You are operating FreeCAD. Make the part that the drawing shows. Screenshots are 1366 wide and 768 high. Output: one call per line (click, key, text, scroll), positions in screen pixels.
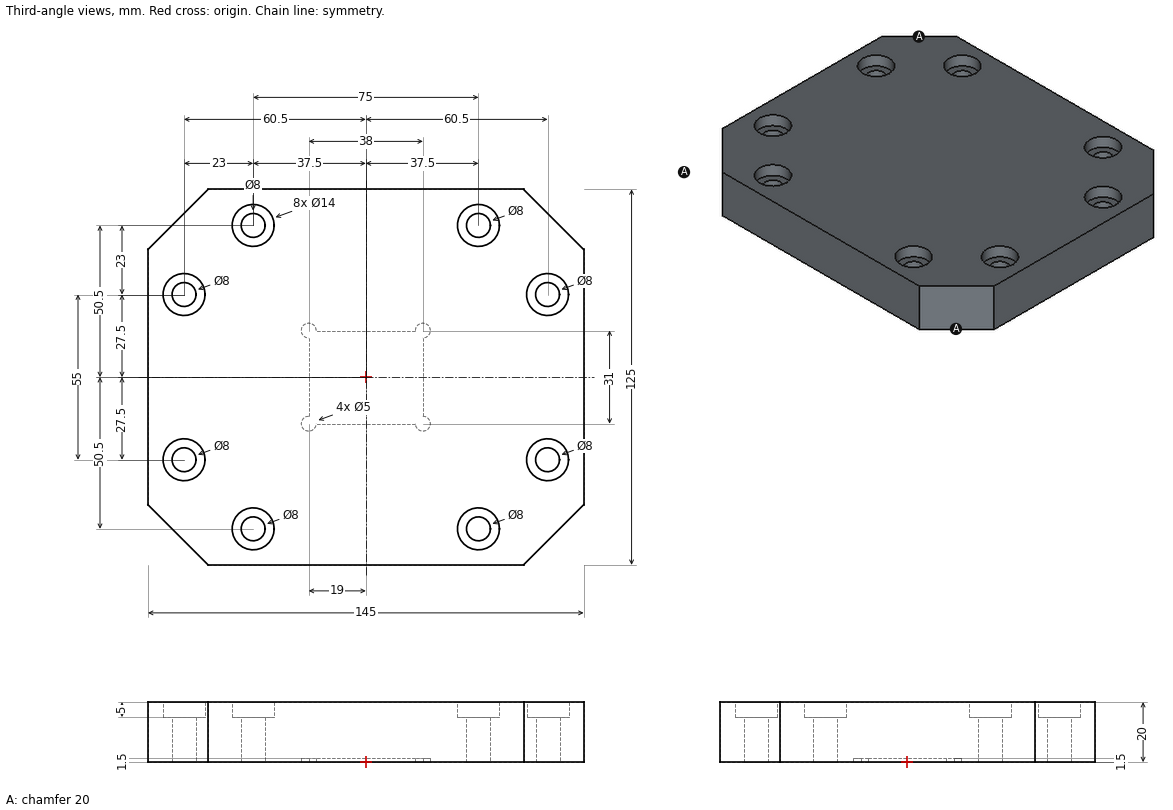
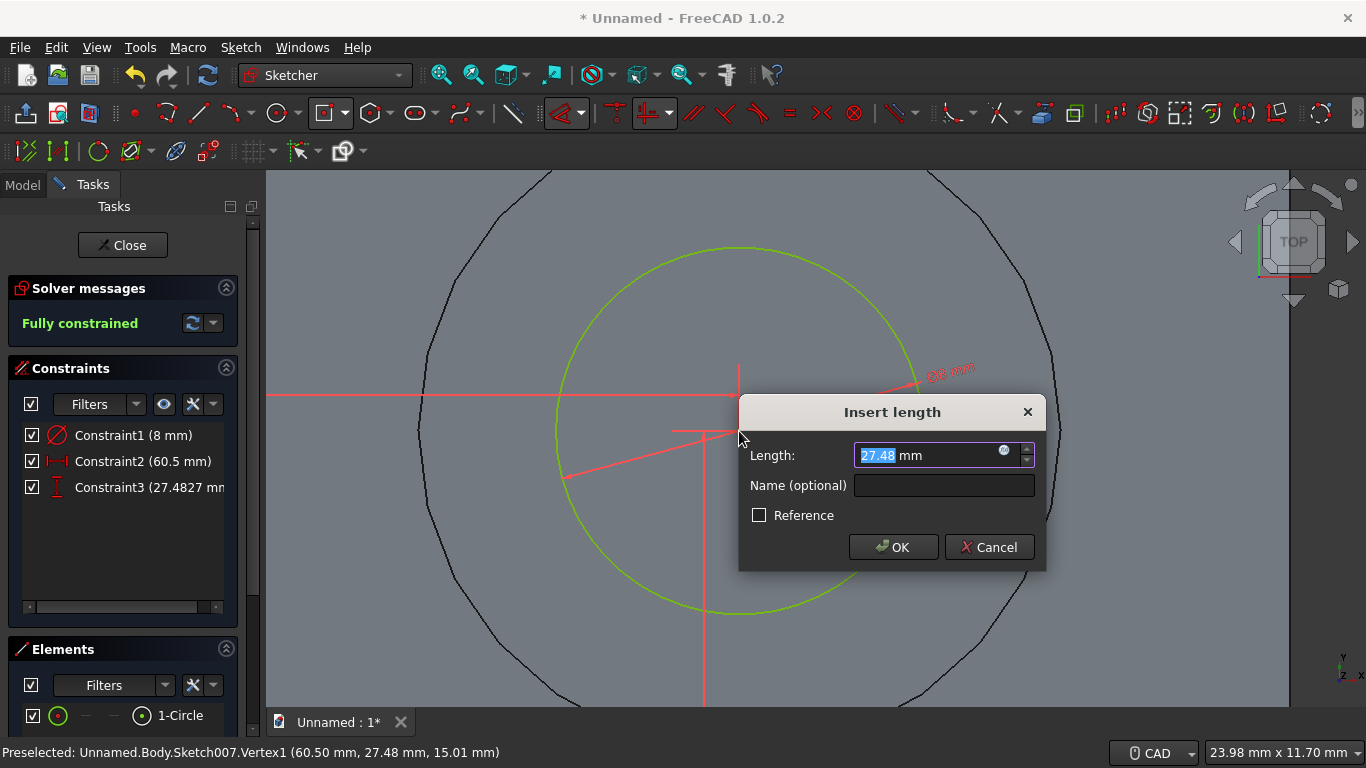
text(27.5)
key(Return)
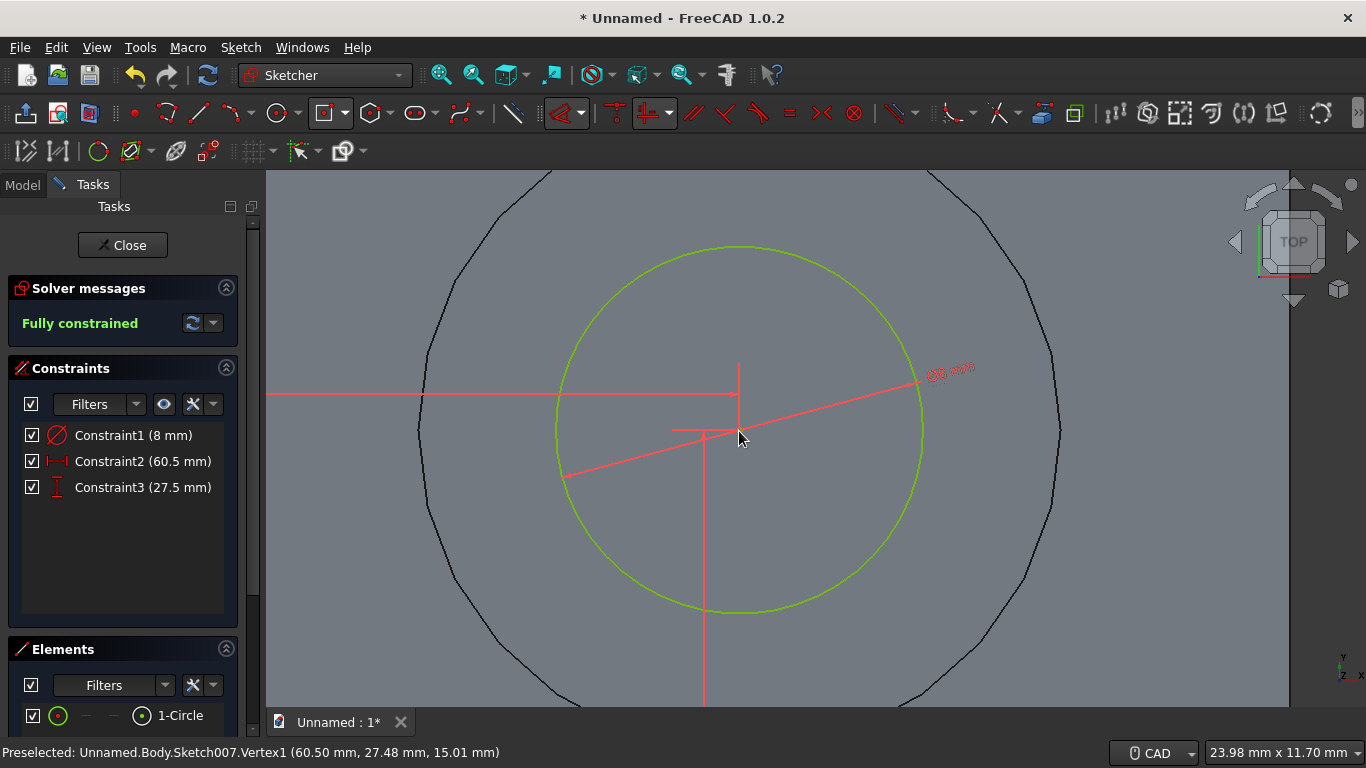
click(123, 245)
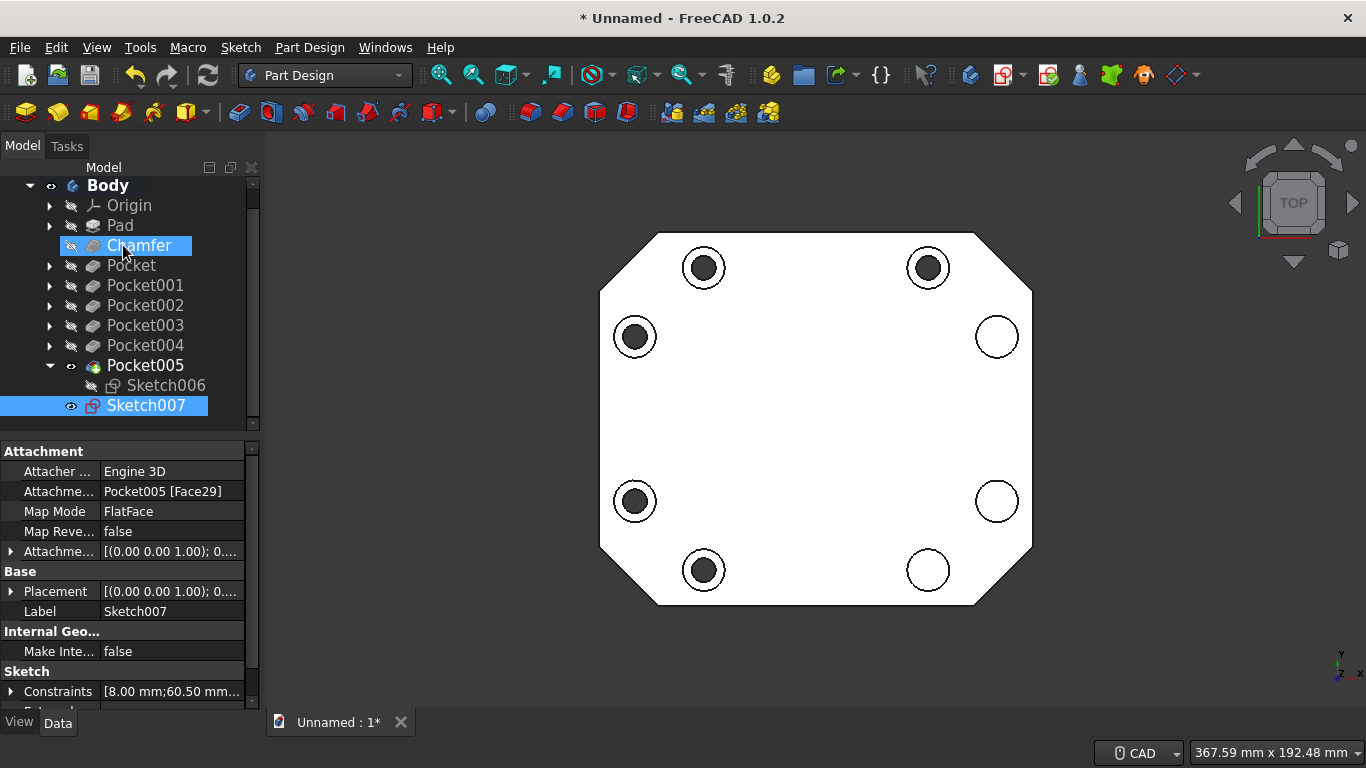
click(240, 112)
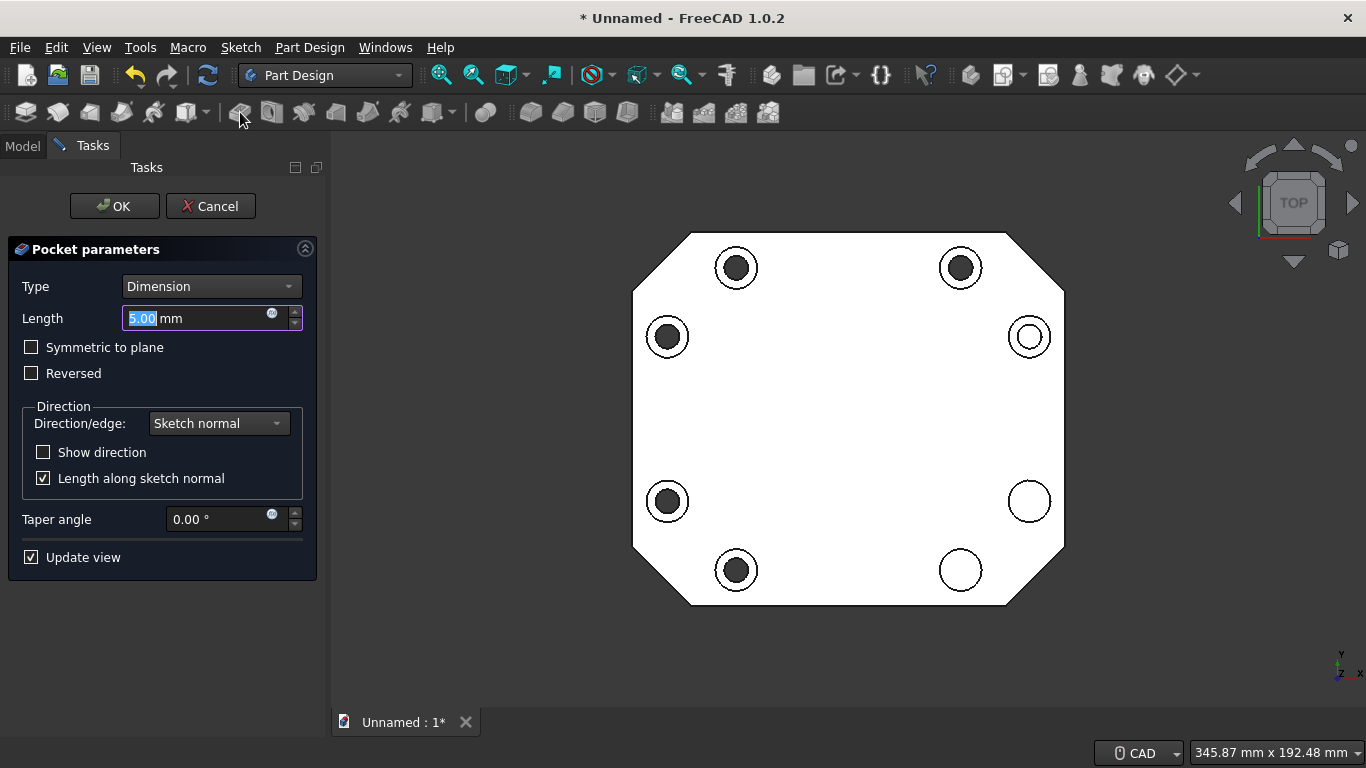
click(212, 286)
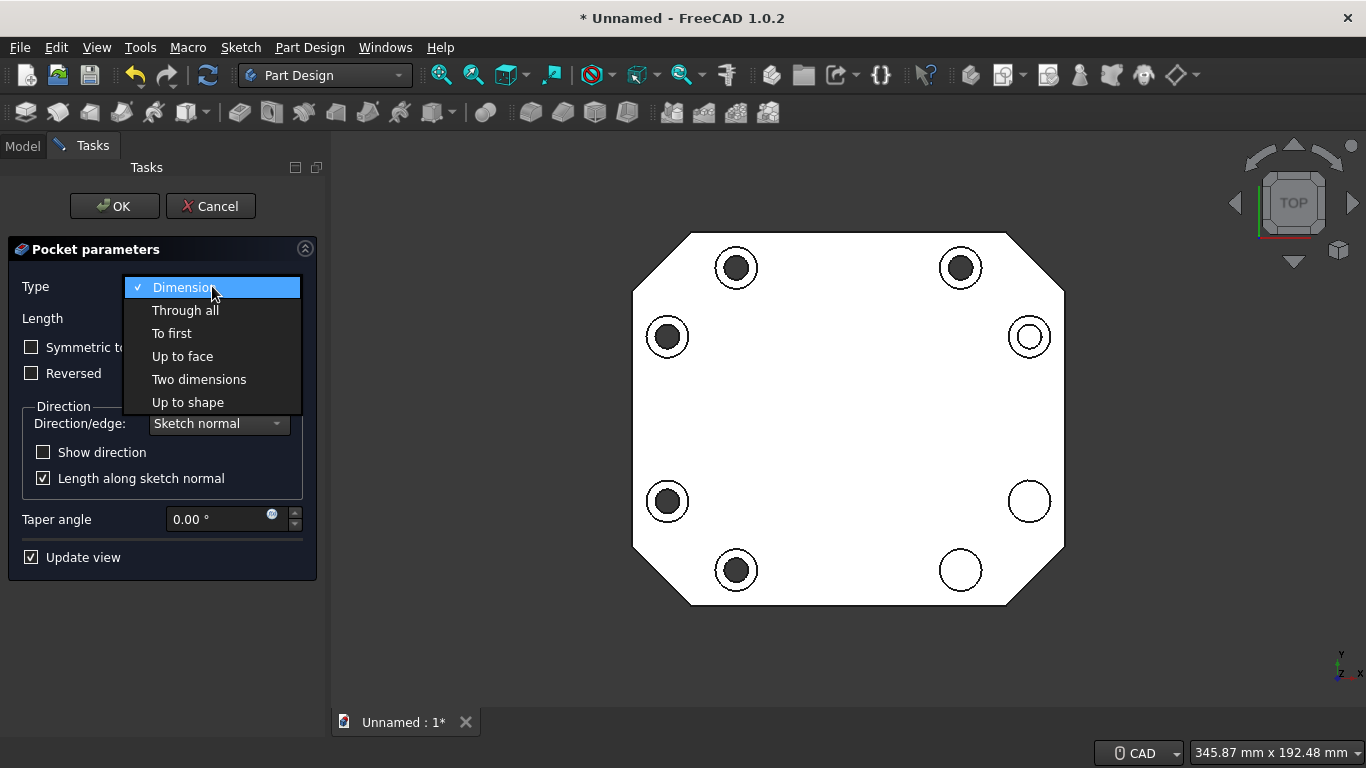
click(212, 334)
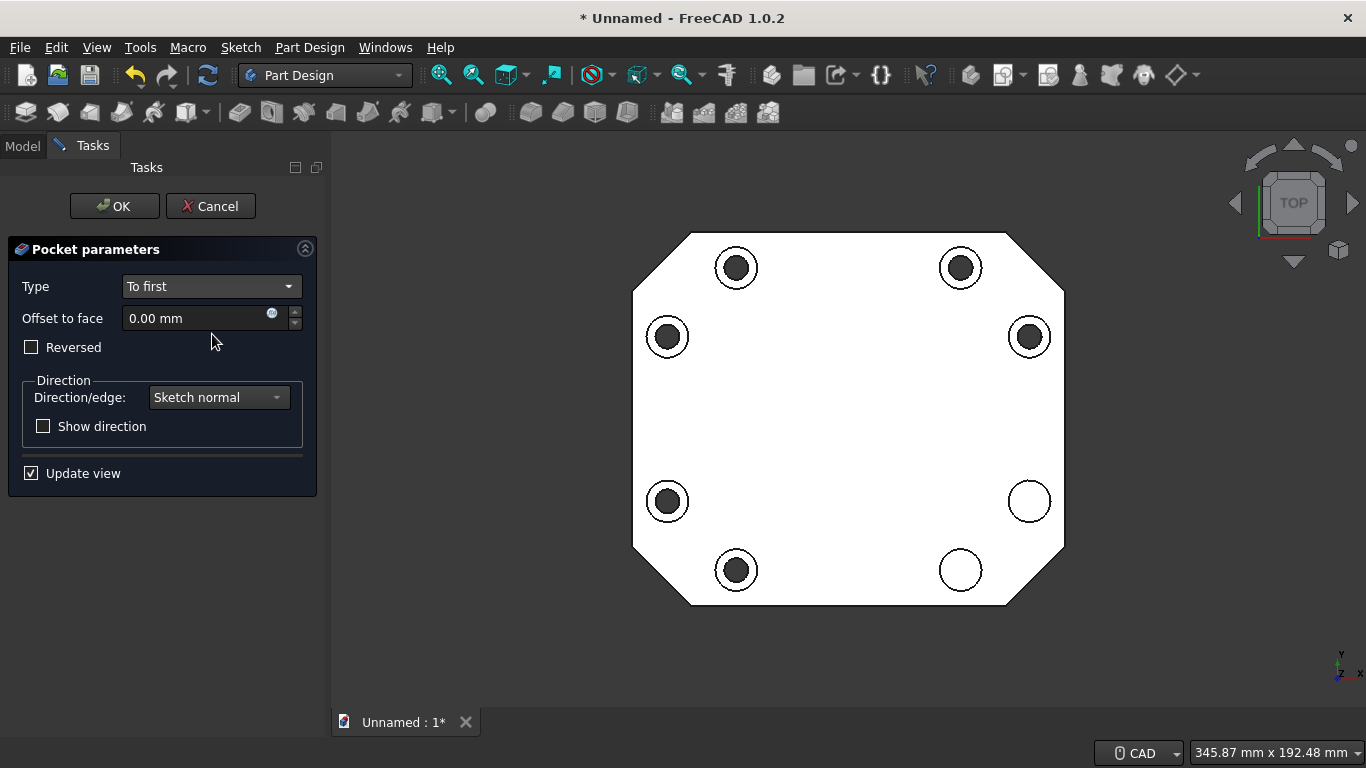
click(115, 206)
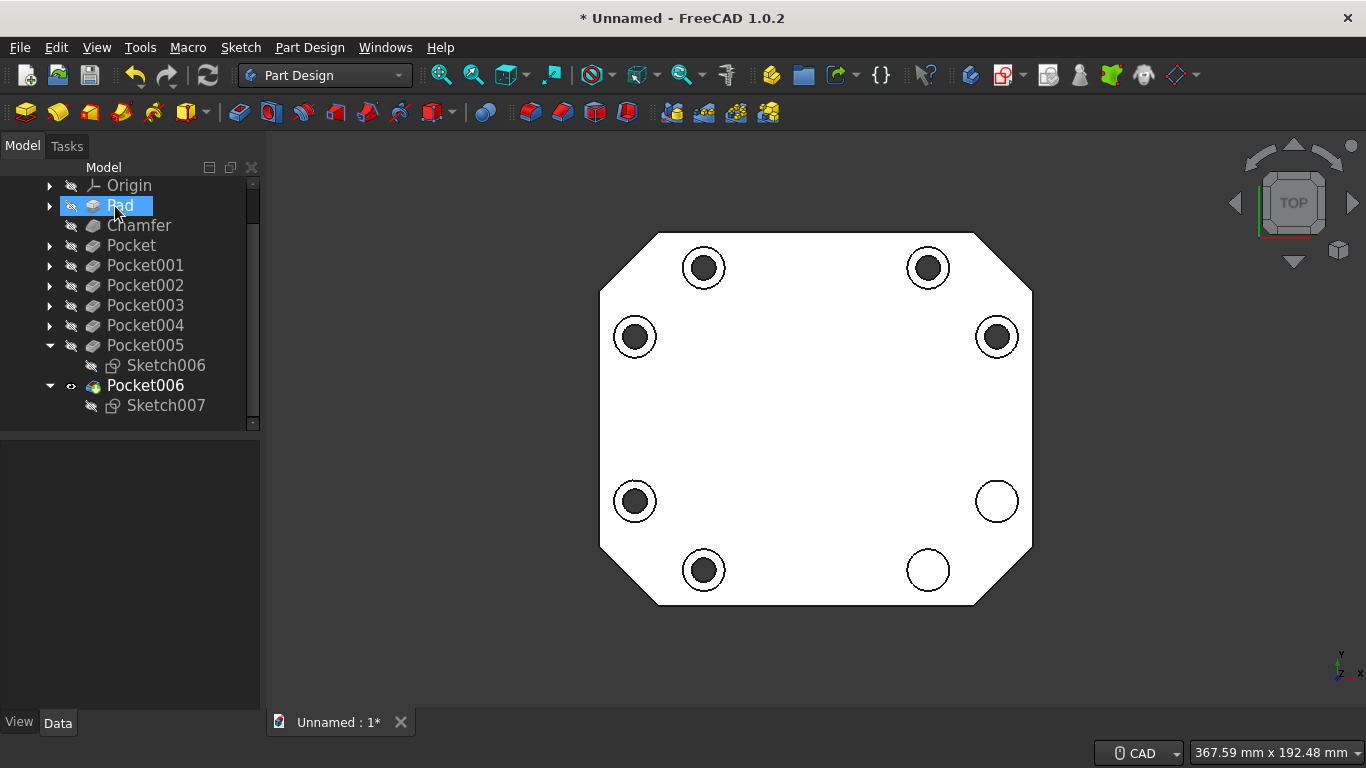
click(928, 569)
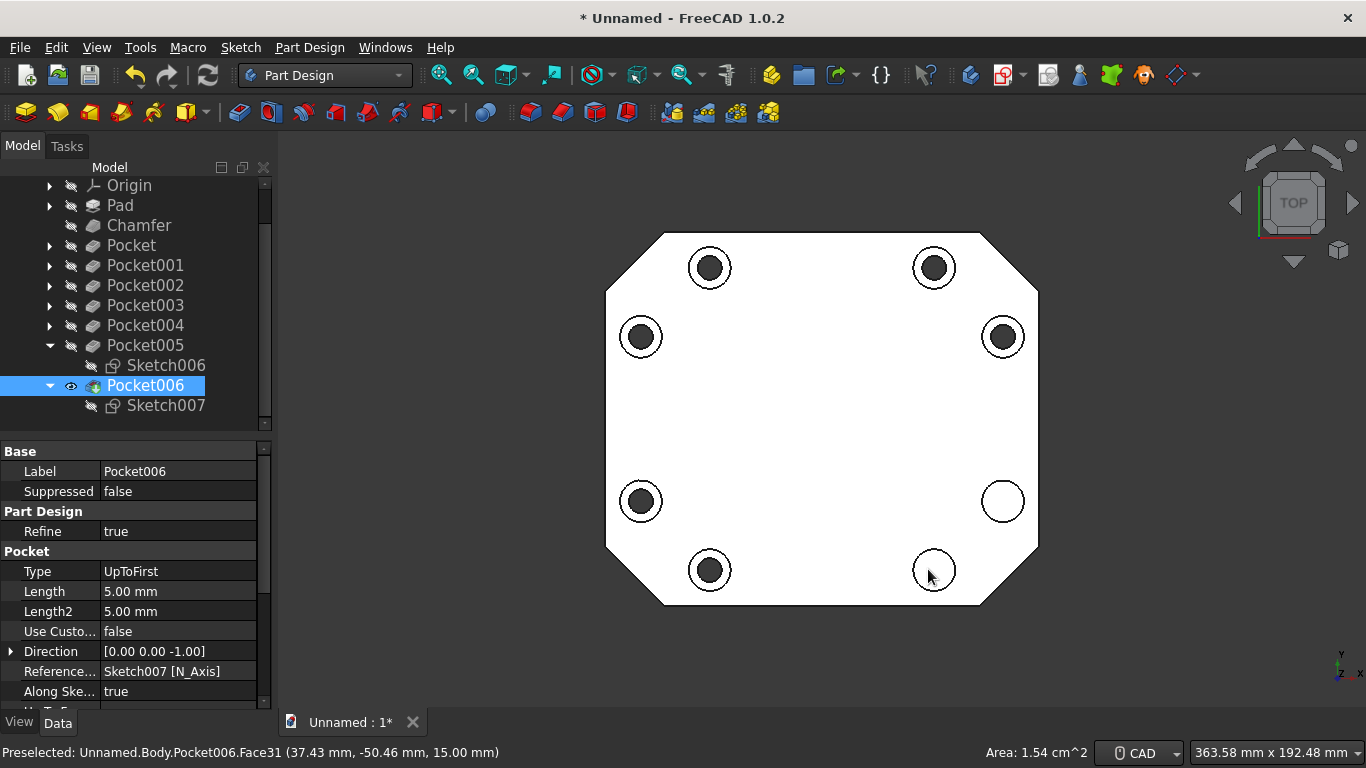
click(1004, 76)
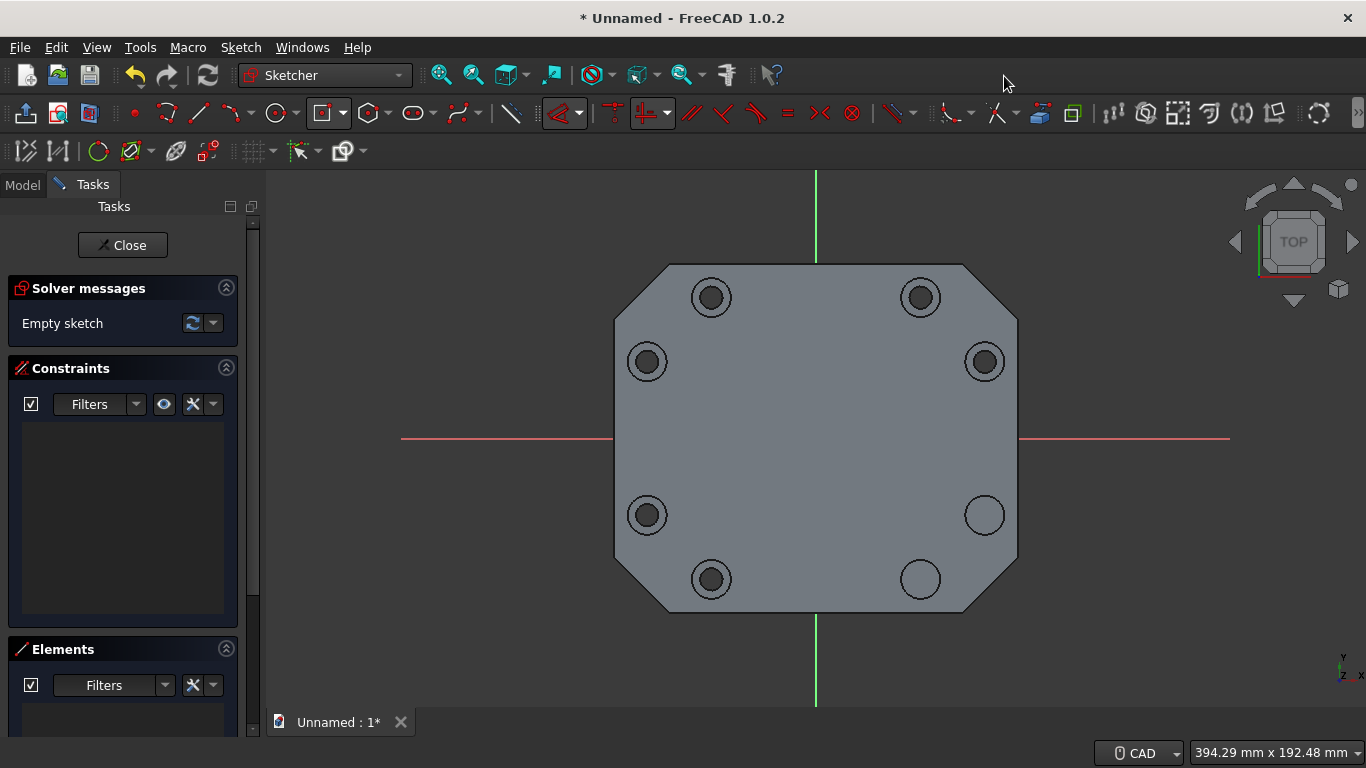
click(90, 114)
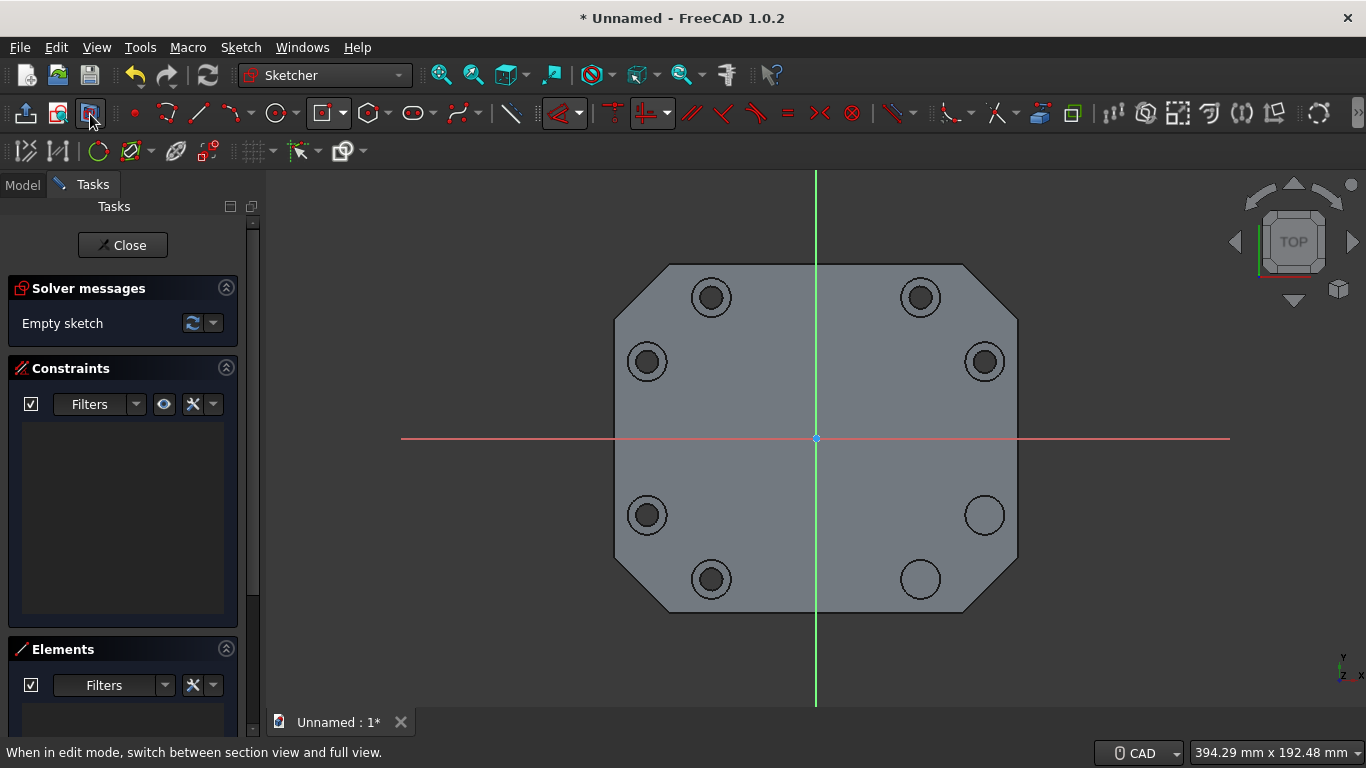
scroll(1000, 520, up, 14)